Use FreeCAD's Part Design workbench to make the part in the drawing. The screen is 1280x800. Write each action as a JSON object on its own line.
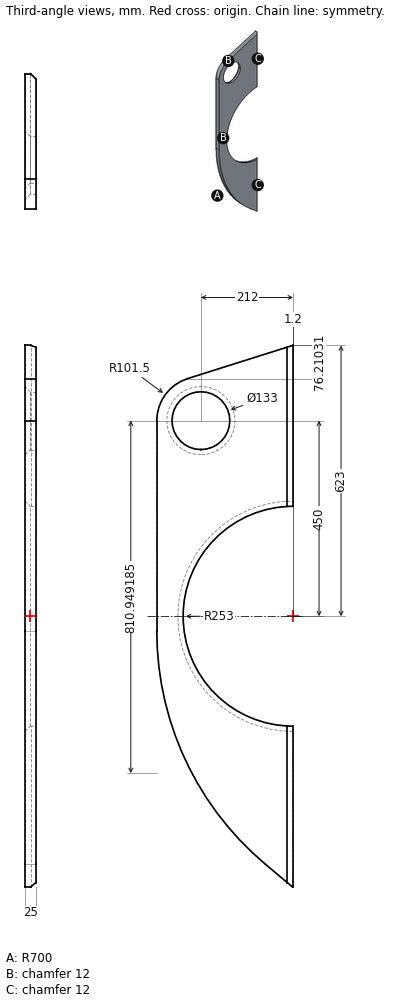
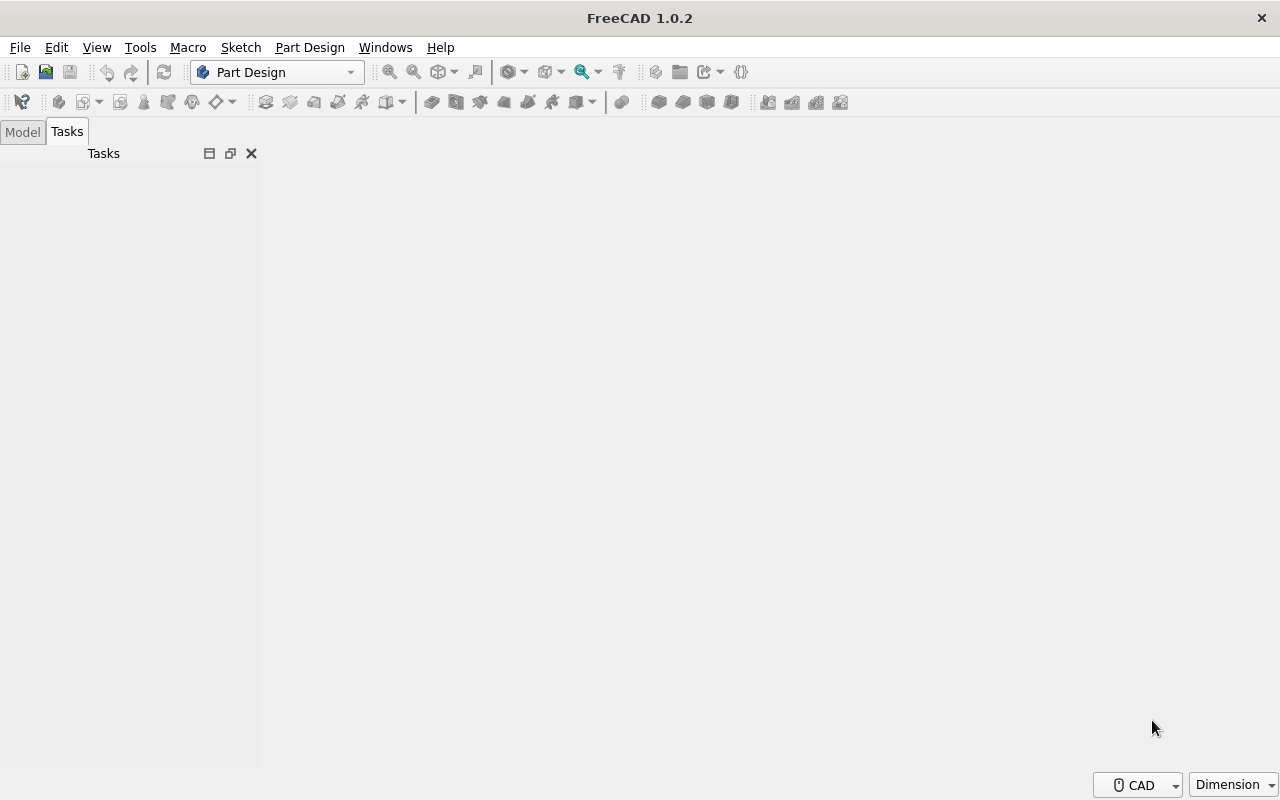
{"action": "left_click", "coordinate": [22, 72]}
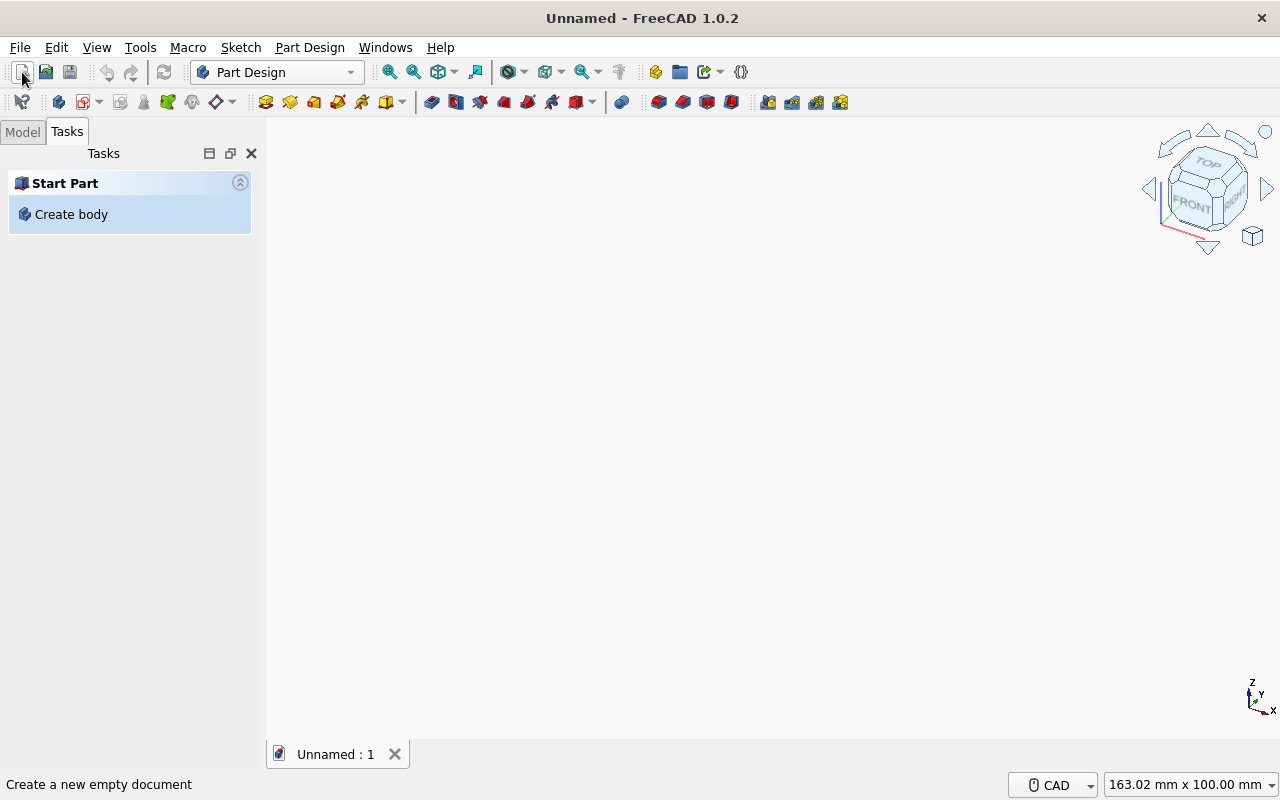
{"action": "left_click", "coordinate": [84, 102]}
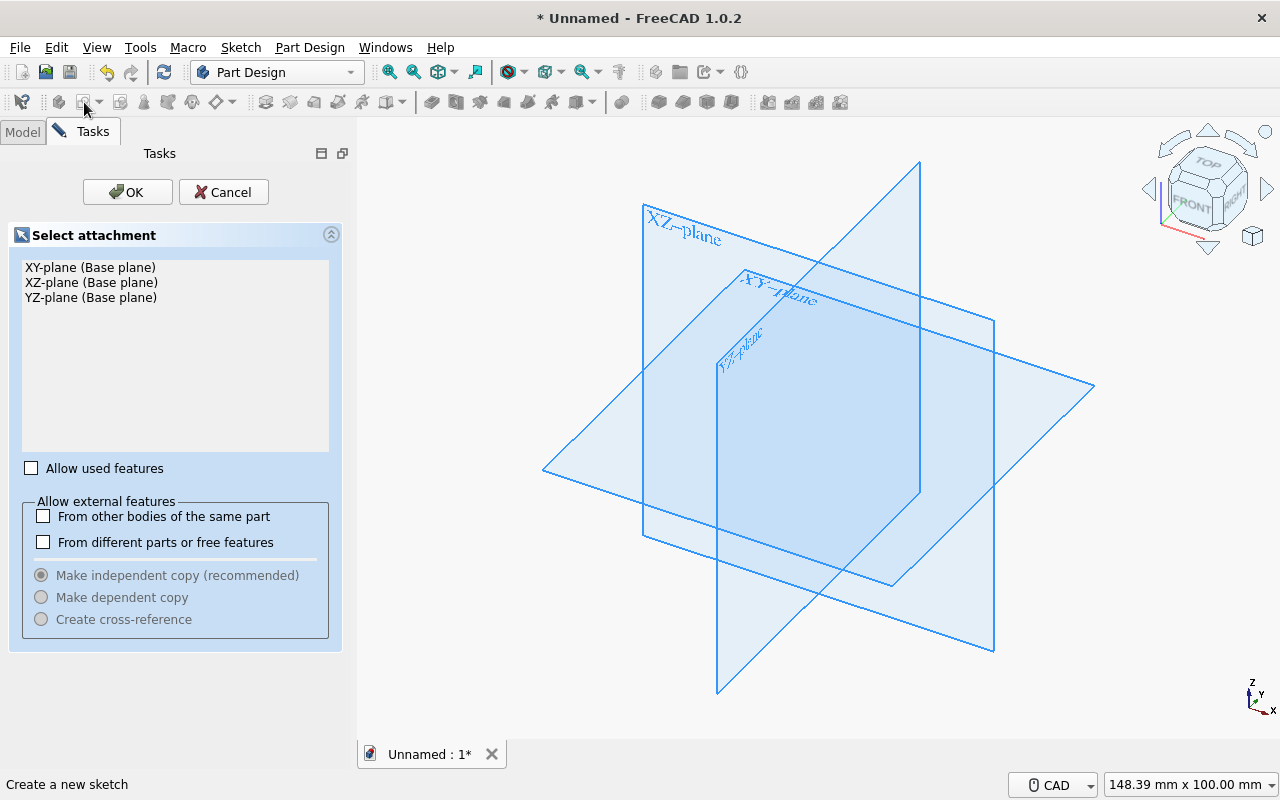
{"action": "left_click", "coordinate": [82, 298]}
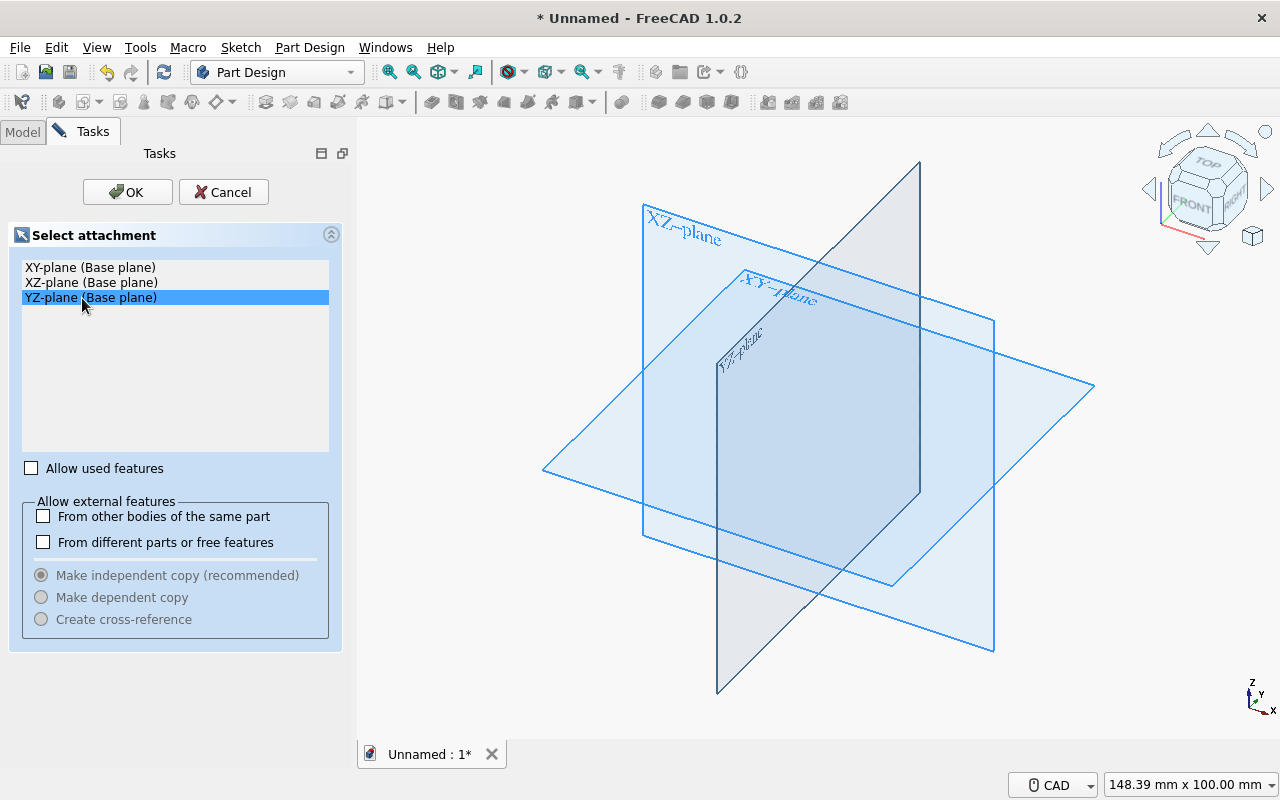
{"action": "left_click", "coordinate": [128, 192]}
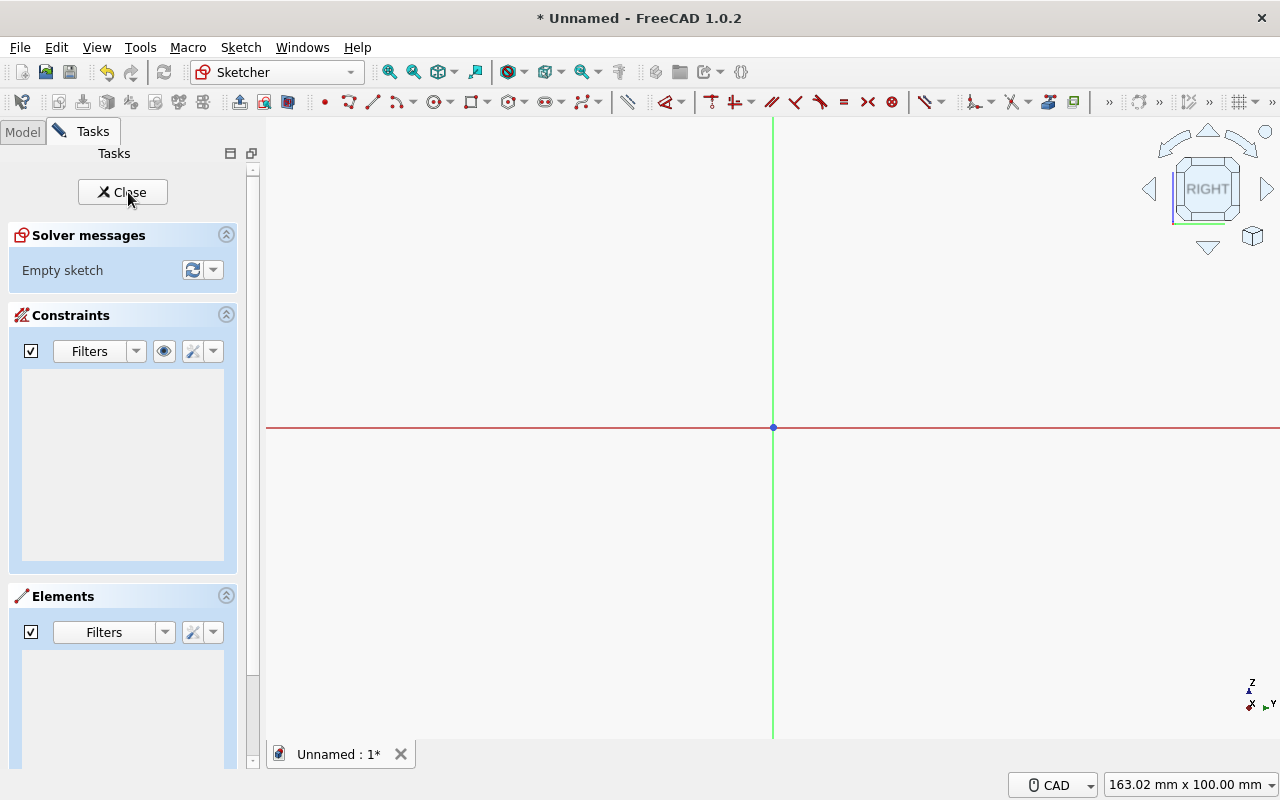
{"action": "scroll", "coordinate": [752, 428], "scroll_direction": "down", "scroll_amount": 15}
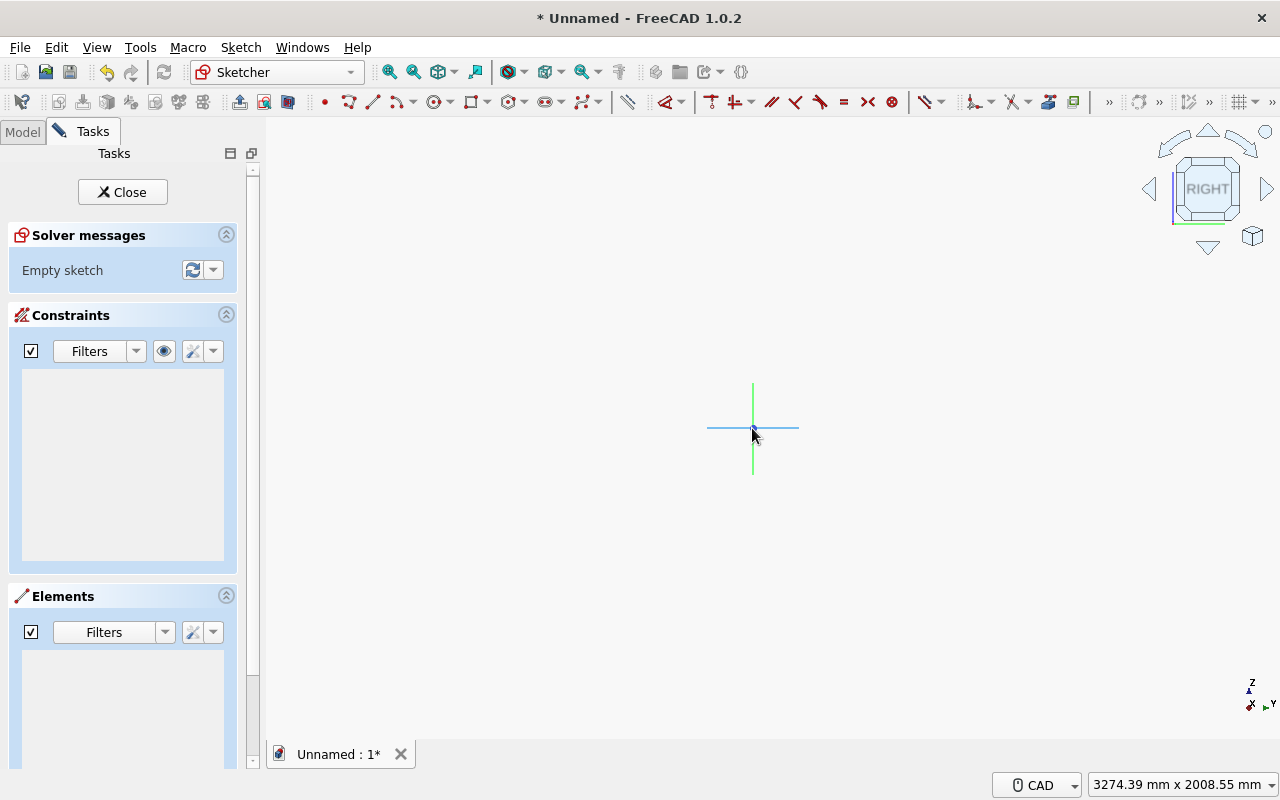
{"action": "left_click", "coordinate": [350, 102]}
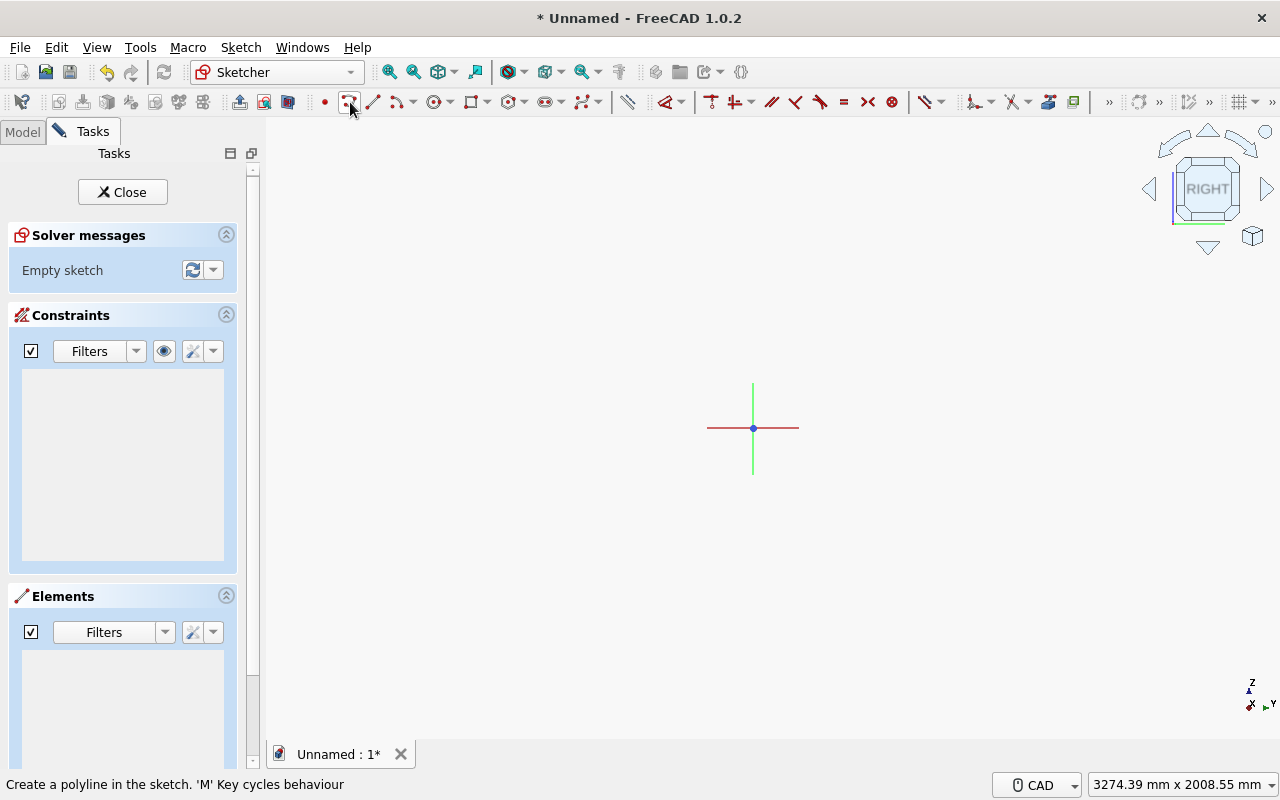
{"action": "scroll", "coordinate": [753, 350], "scroll_direction": "up", "scroll_amount": 19}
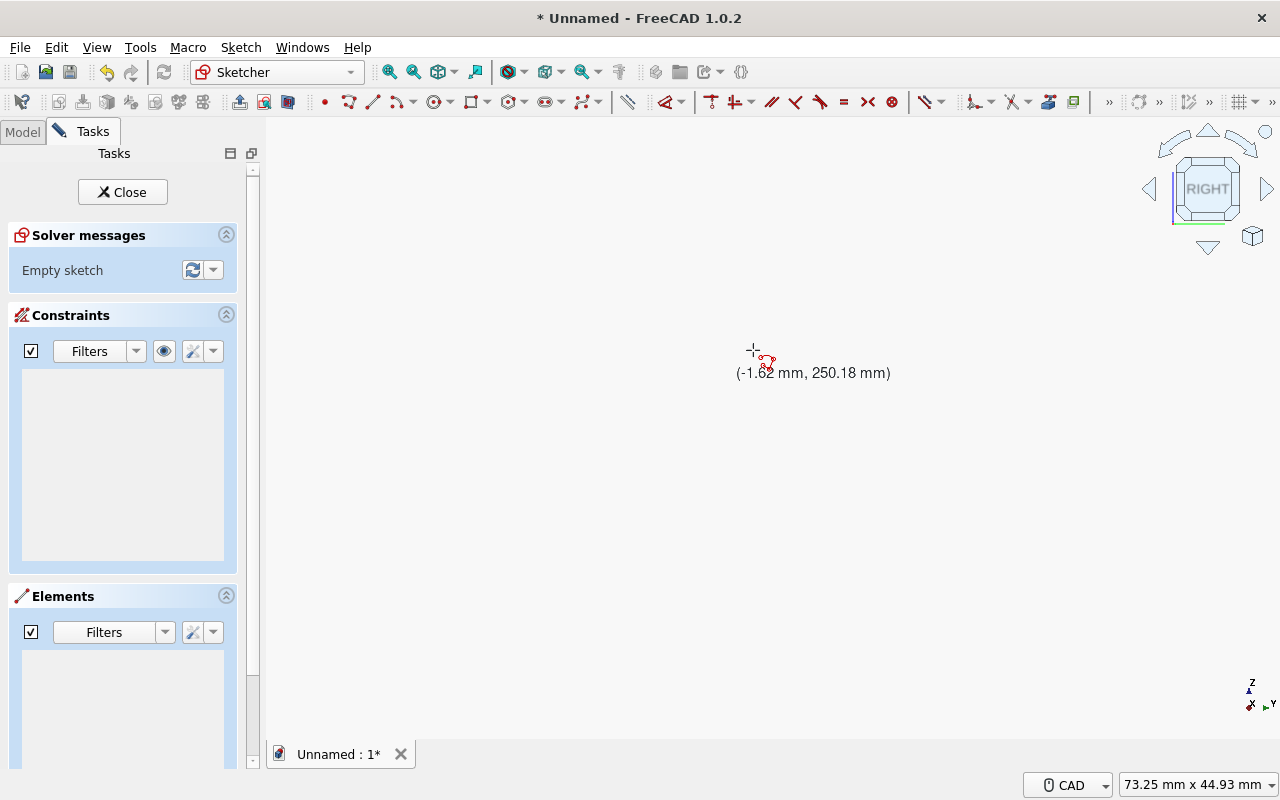
{"action": "left_click", "coordinate": [738, 339]}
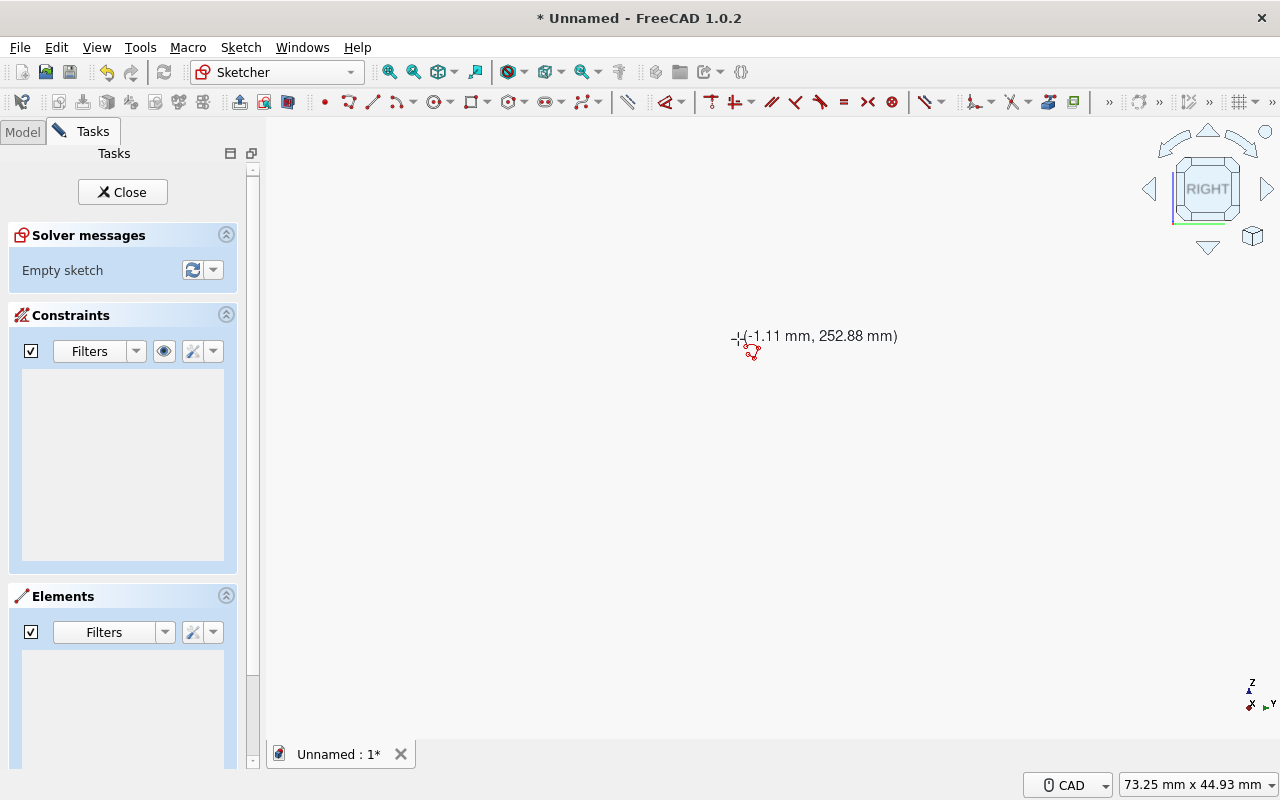
{"action": "scroll", "coordinate": [764, 332], "scroll_direction": "down", "scroll_amount": 18}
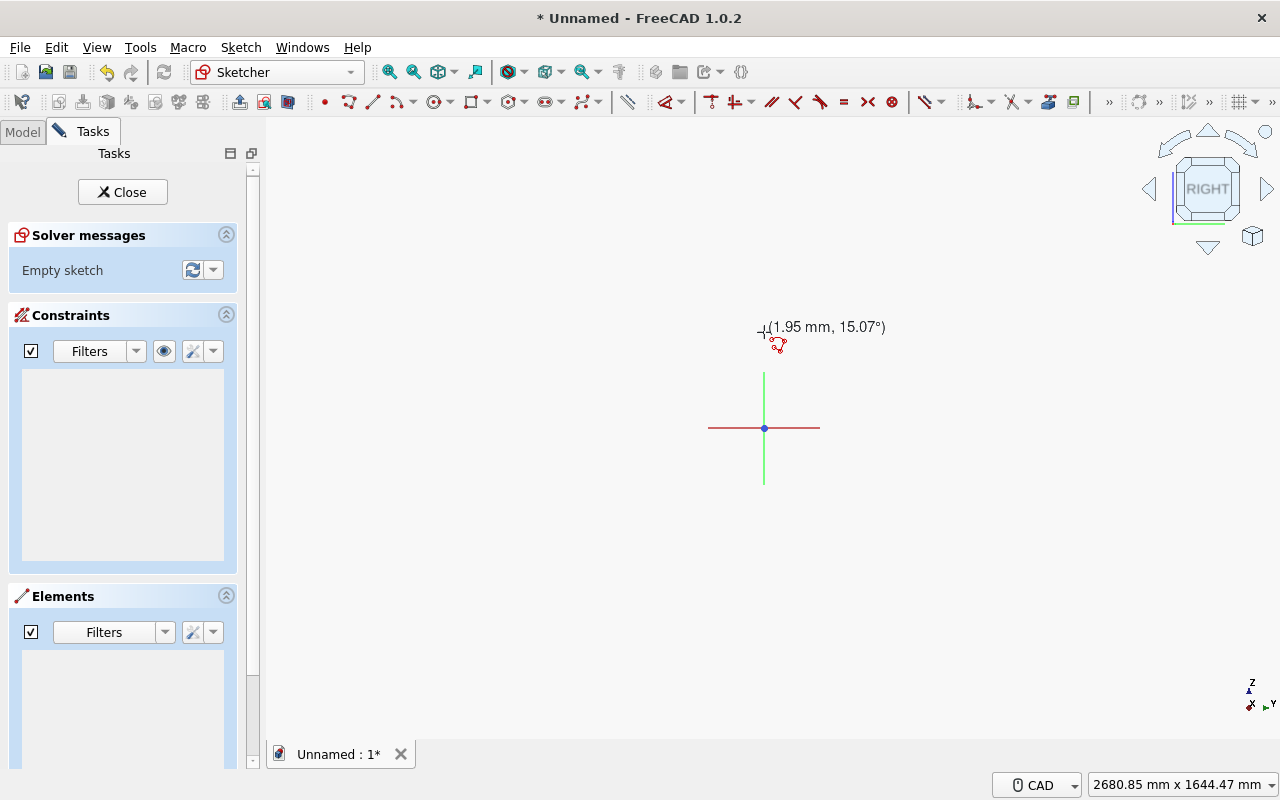
{"action": "scroll", "coordinate": [764, 193], "scroll_direction": "up", "scroll_amount": 18}